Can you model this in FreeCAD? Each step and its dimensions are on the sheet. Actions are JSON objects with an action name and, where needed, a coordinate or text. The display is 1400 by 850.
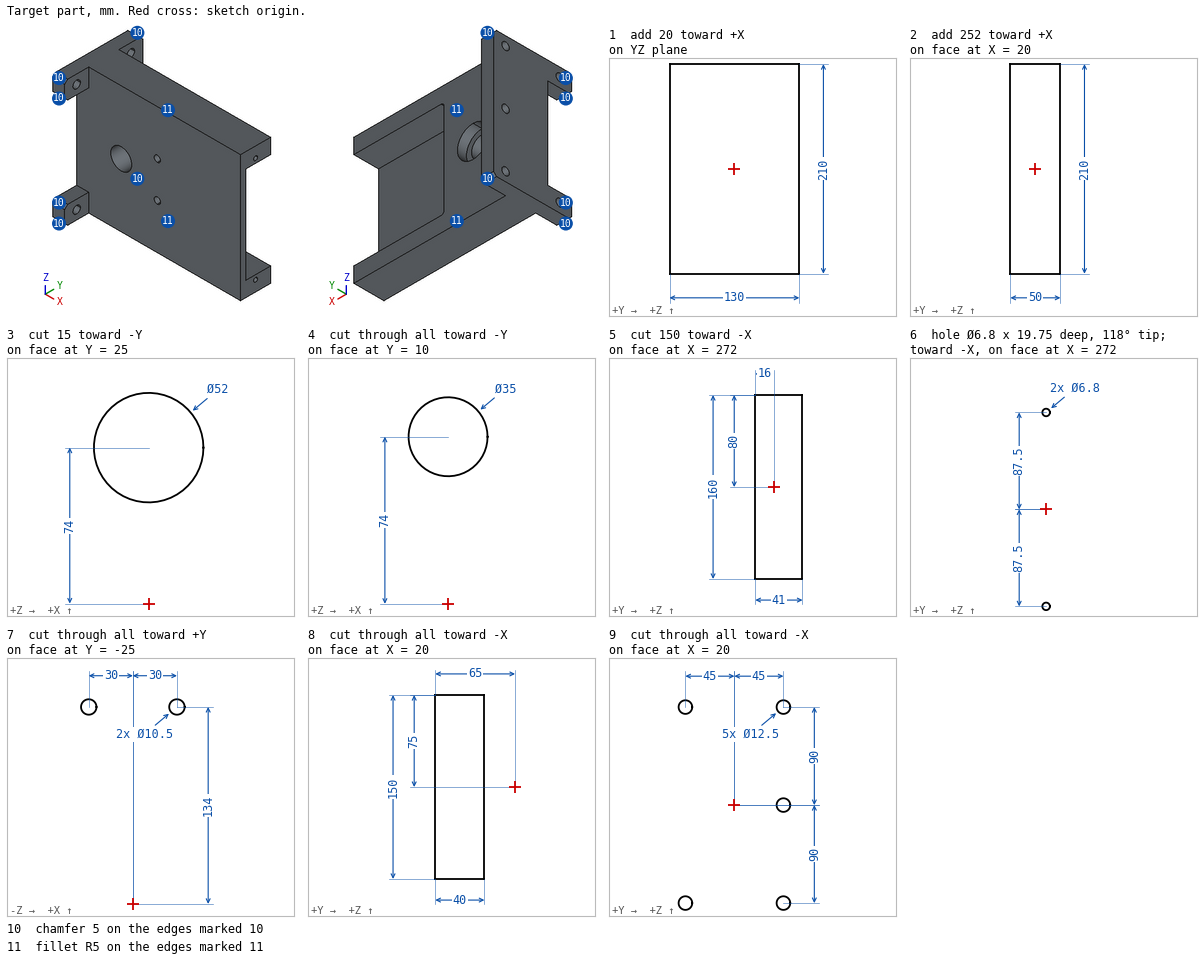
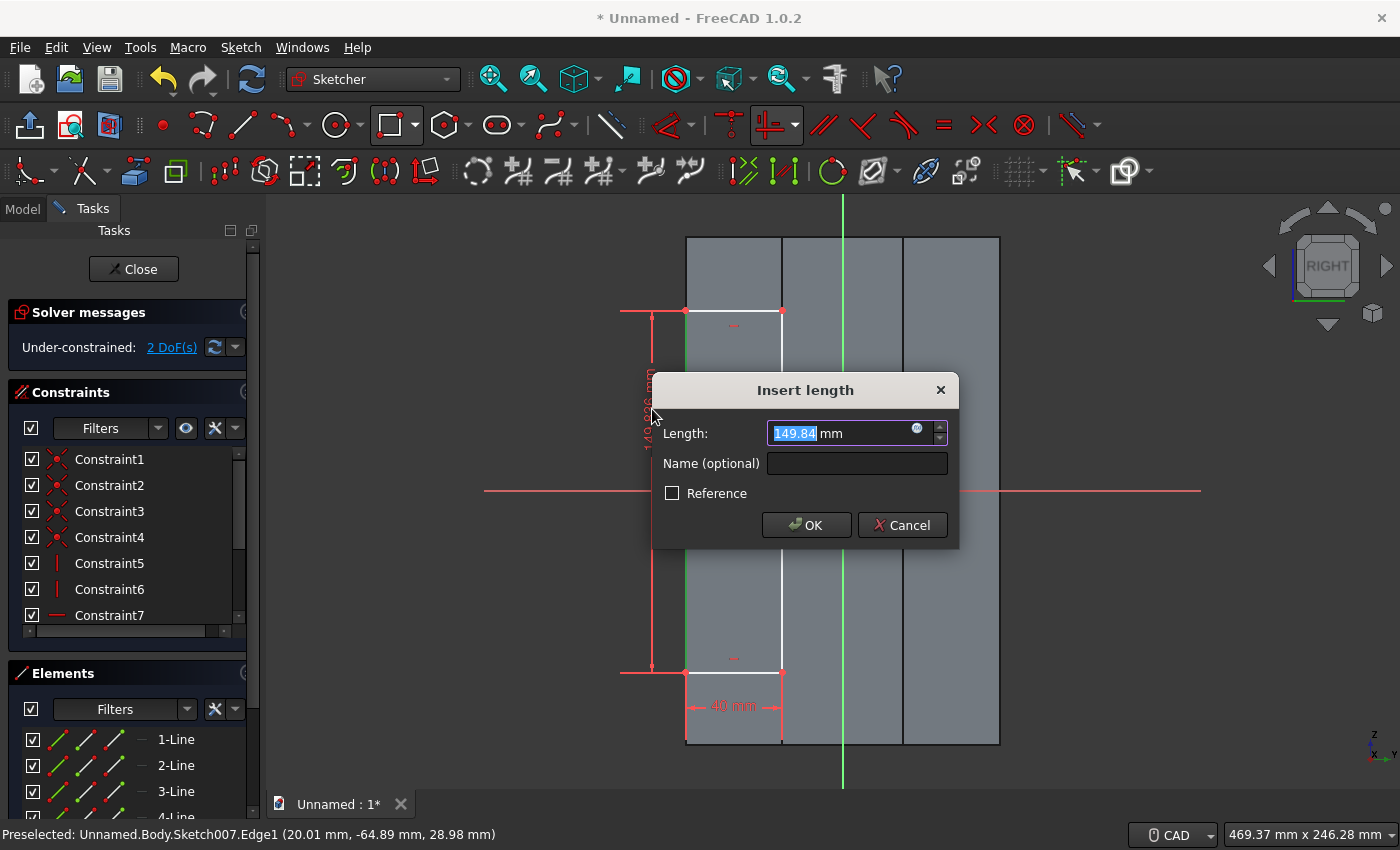
{"action": "type", "text": "150"}
{"action": "key", "text": "Return"}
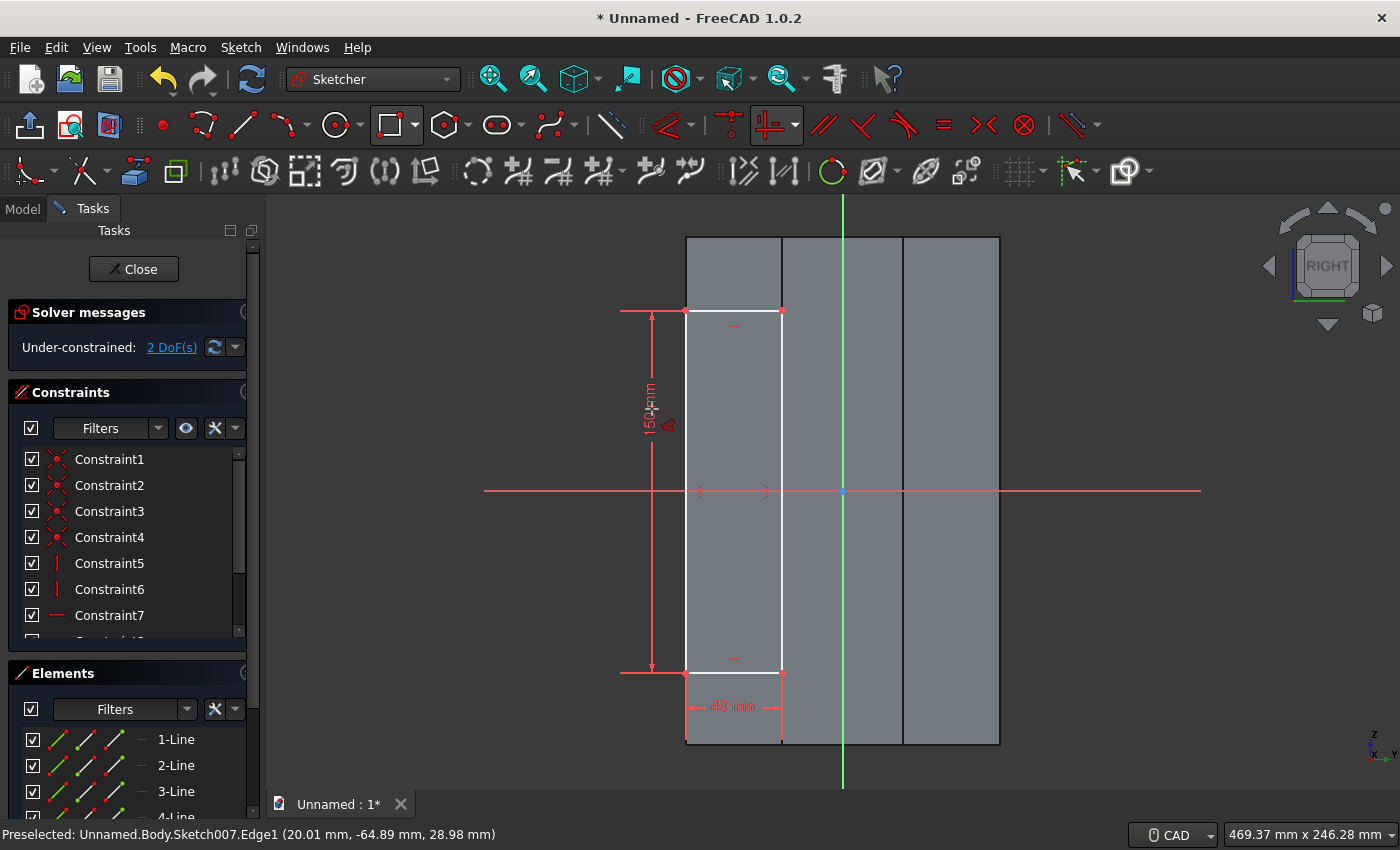
{"action": "left_click", "coordinate": [686, 311]}
{"action": "left_click", "coordinate": [764, 277]}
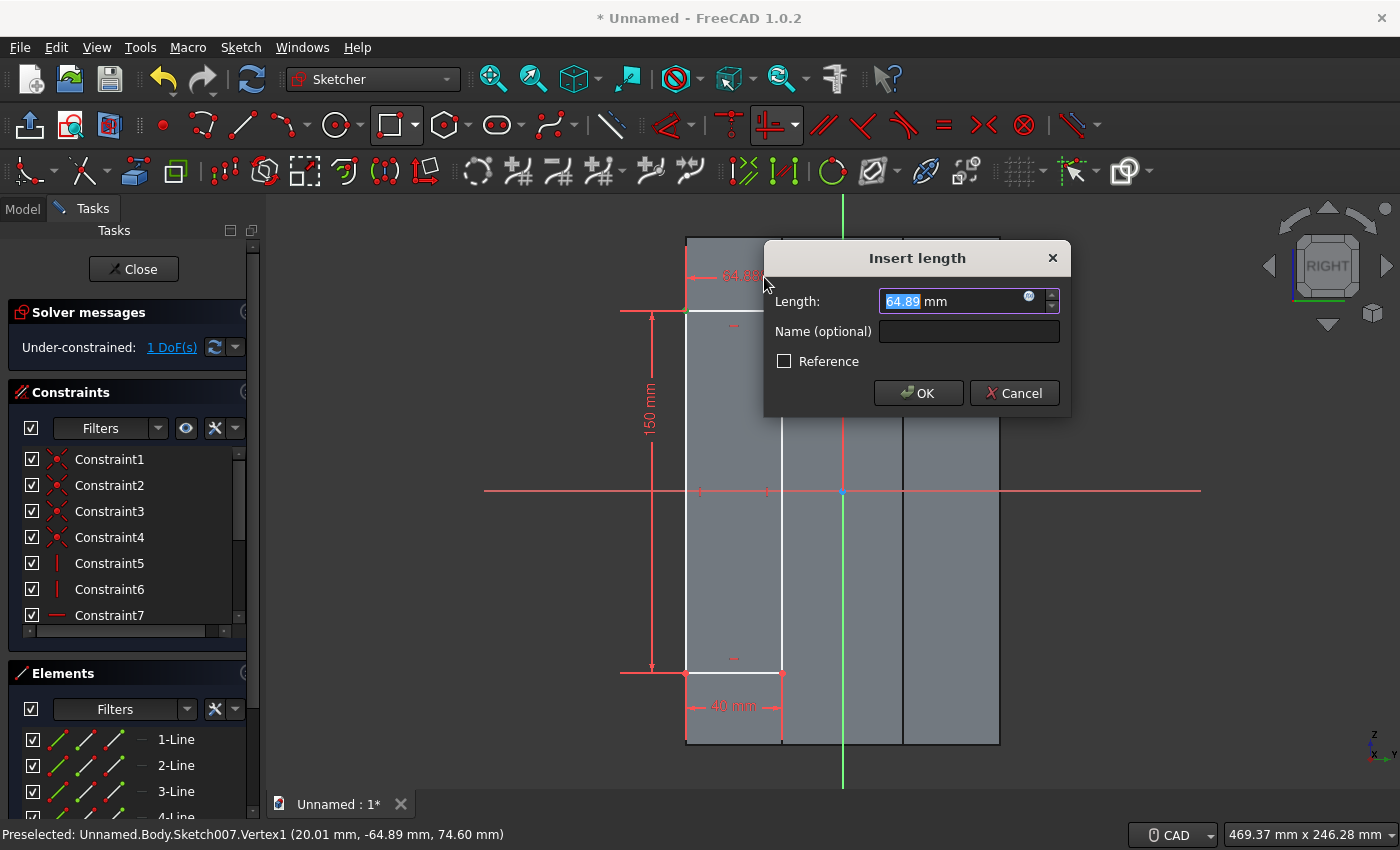
{"action": "type", "text": "65"}
{"action": "key", "text": "Return"}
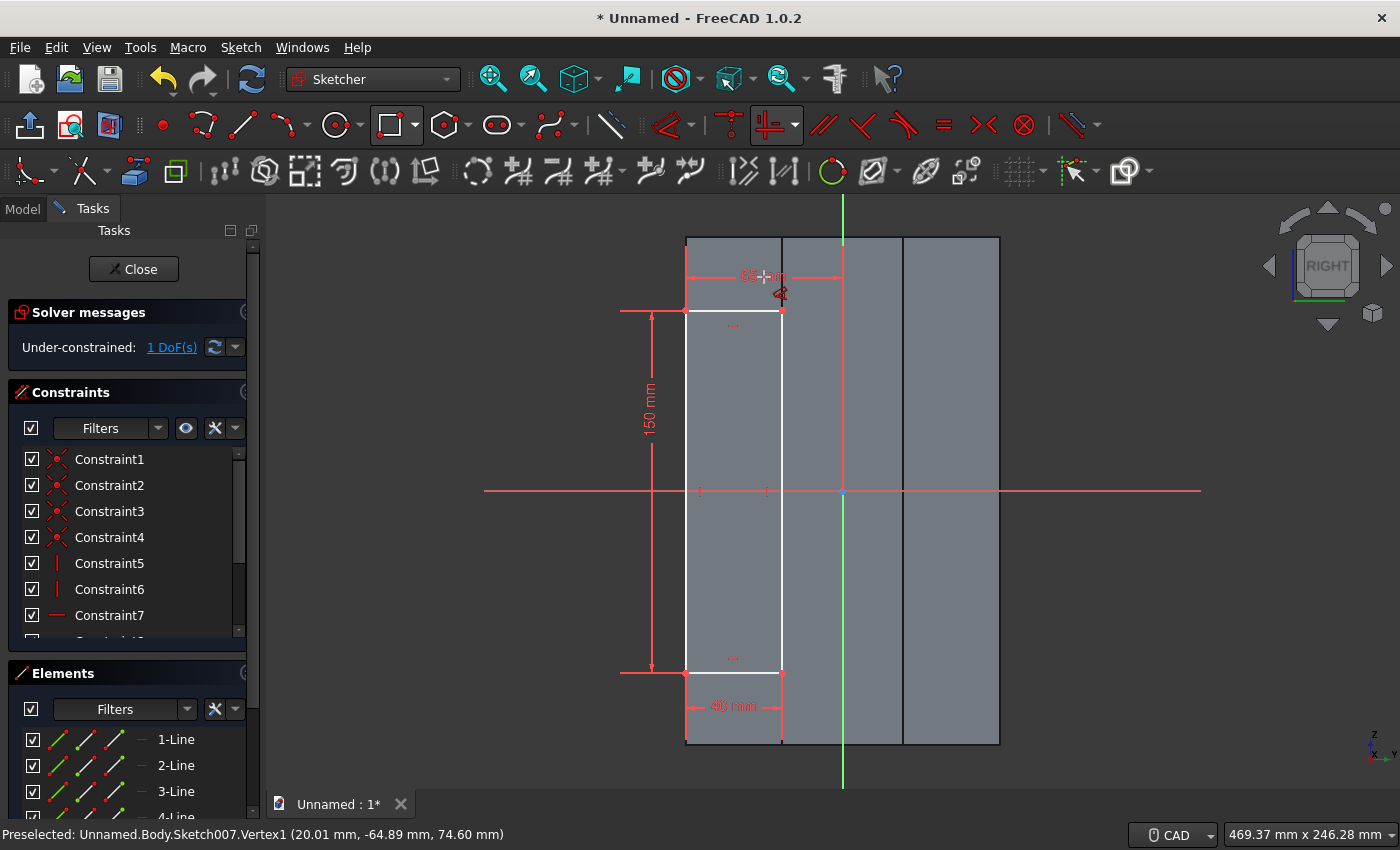
{"action": "left_click", "coordinate": [686, 311]}
{"action": "left_click", "coordinate": [877, 401]}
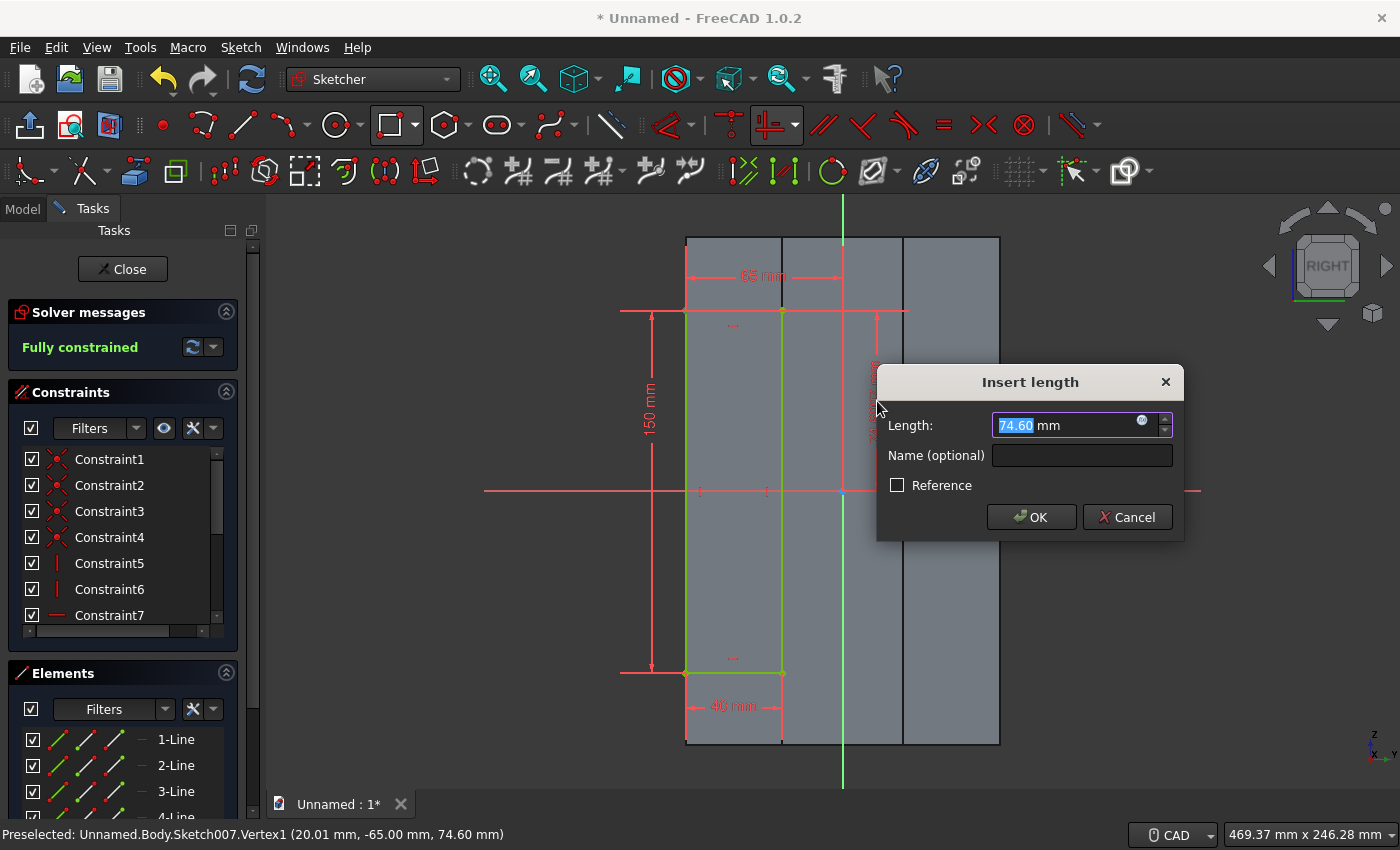
{"action": "type", "text": "75"}
{"action": "key", "text": "Return"}
{"action": "key", "text": "Escape"}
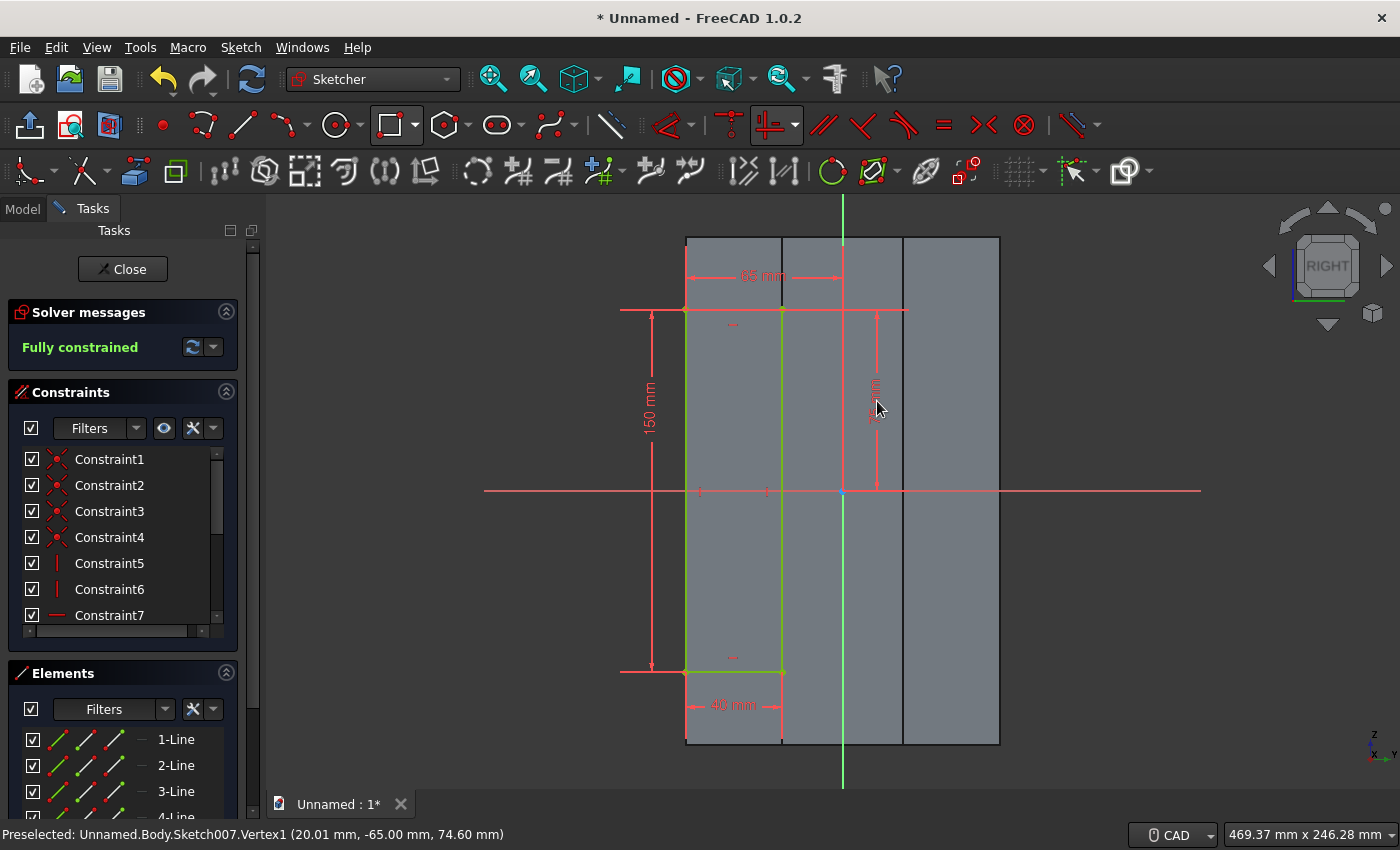
{"action": "left_click", "coordinate": [123, 269]}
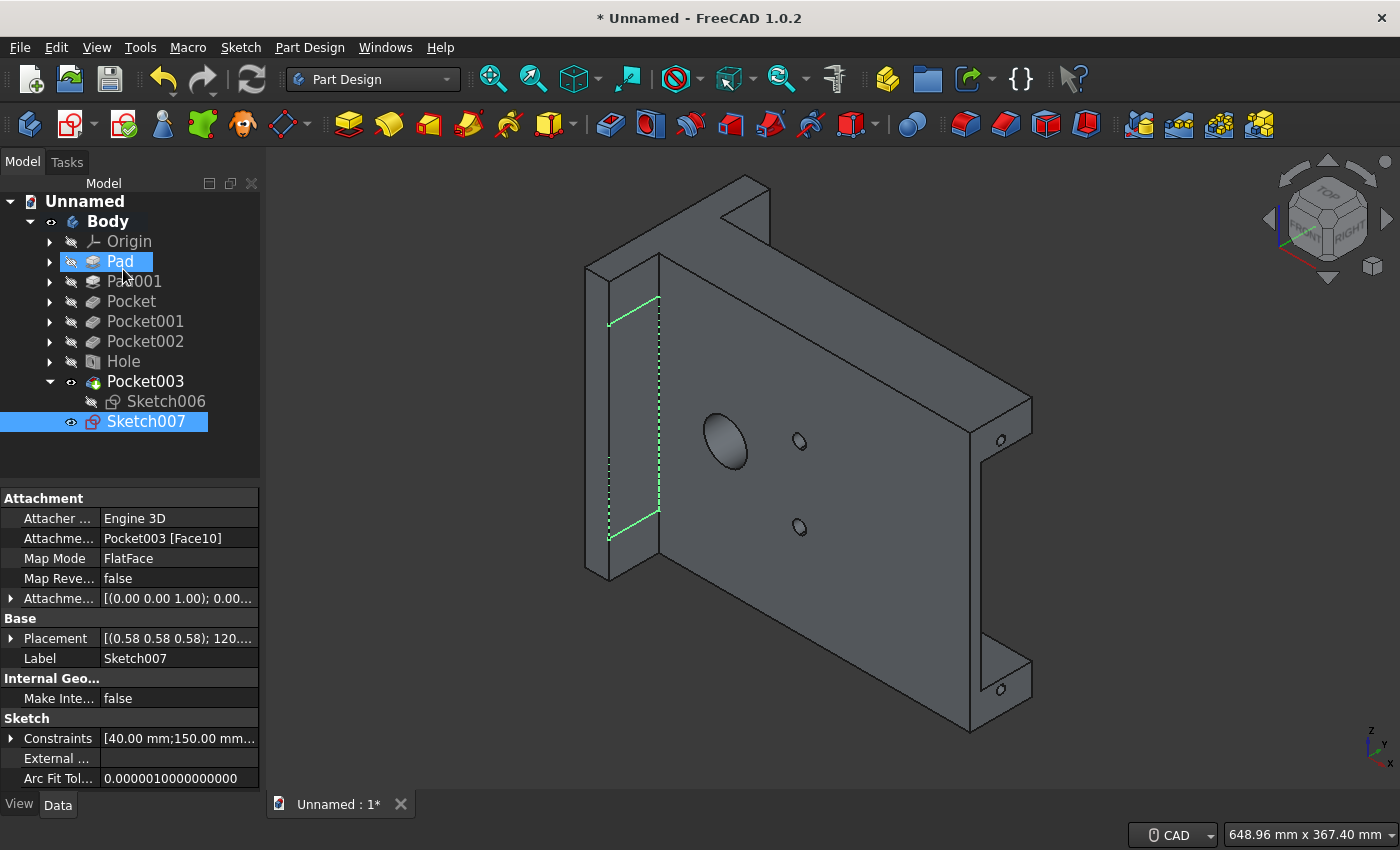
{"action": "left_click", "coordinate": [612, 124]}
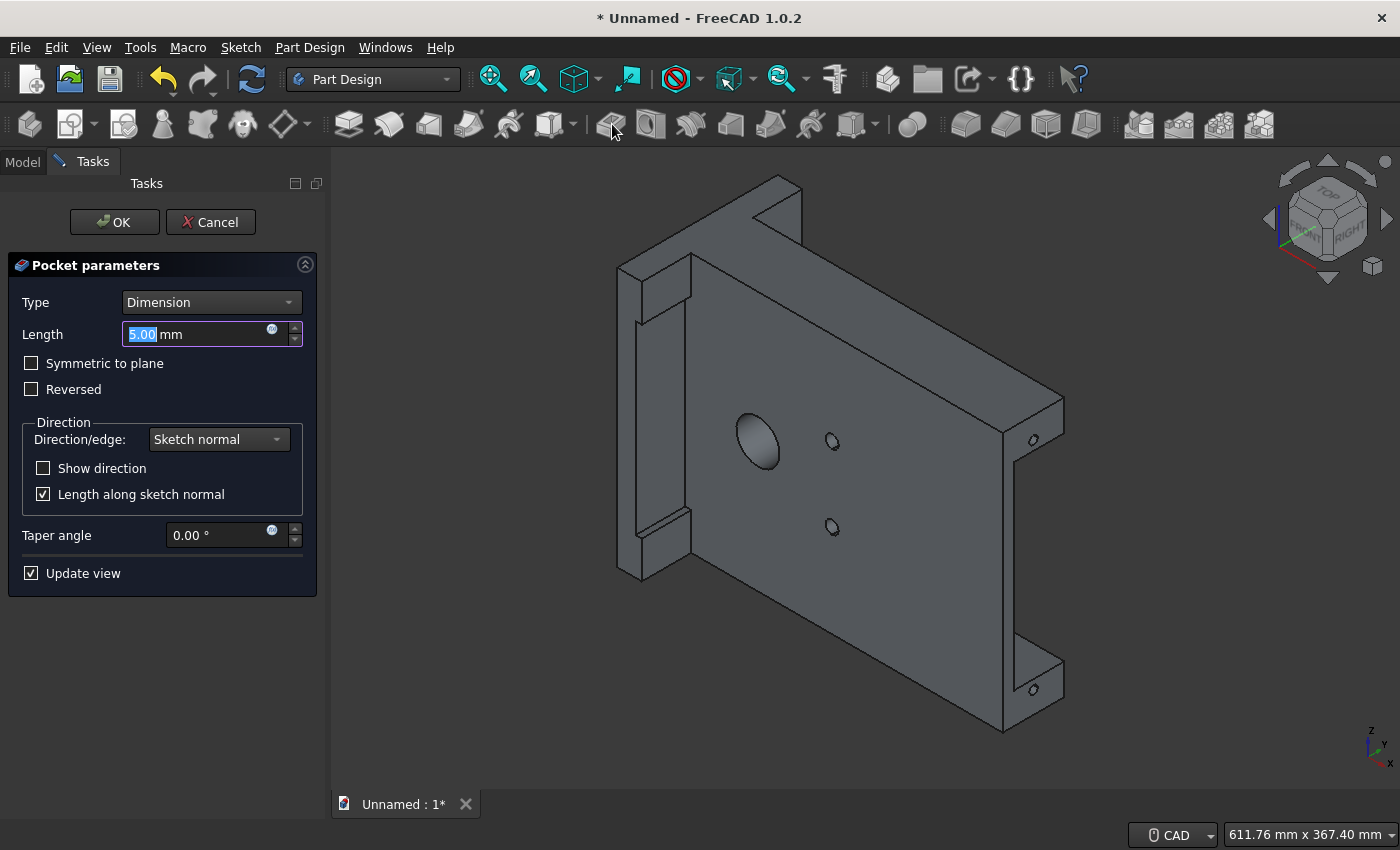
{"action": "left_click", "coordinate": [212, 302]}